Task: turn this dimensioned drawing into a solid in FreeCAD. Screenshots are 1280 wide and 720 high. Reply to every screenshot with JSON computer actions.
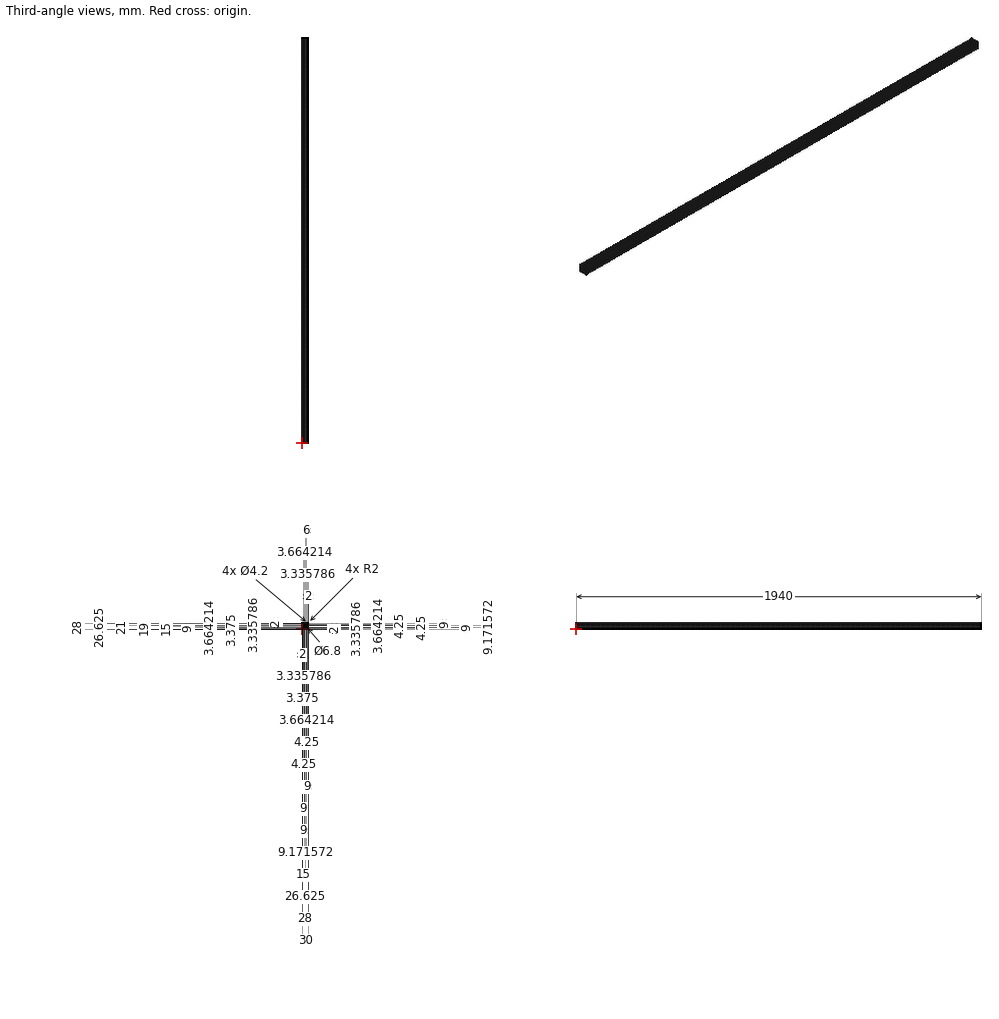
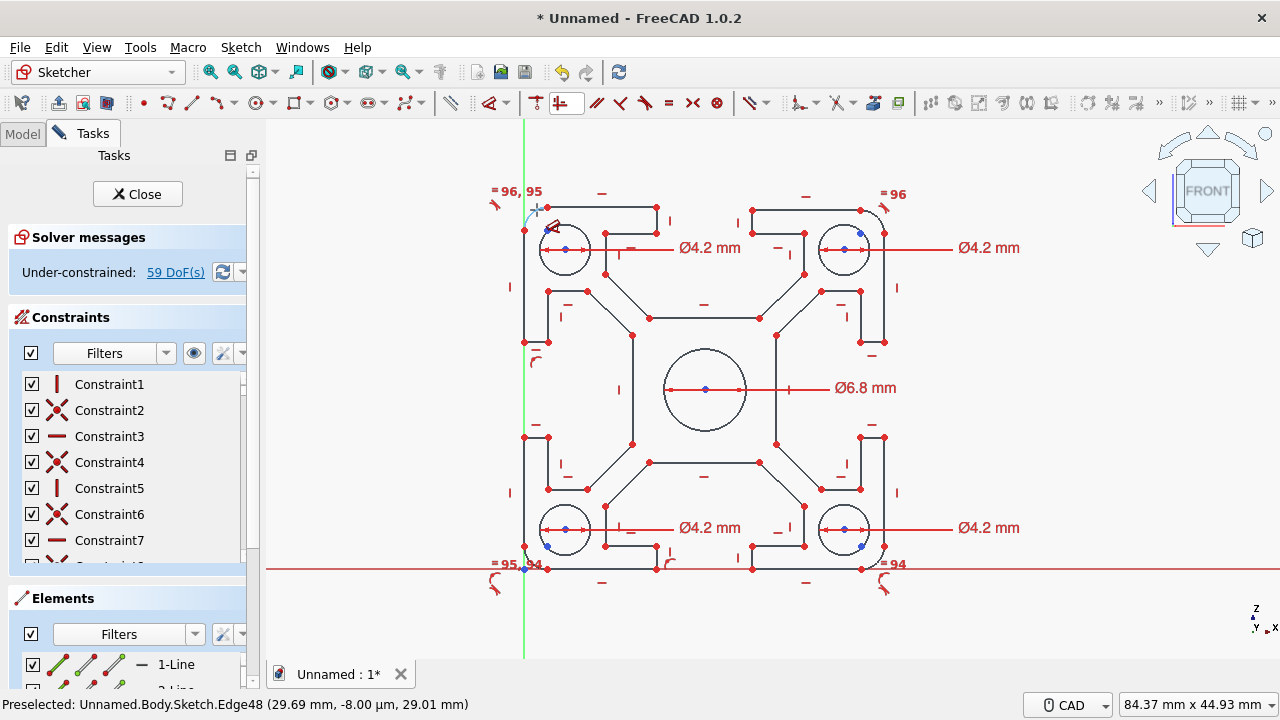
{"action": "scroll", "coordinate": [872, 567], "scroll_direction": "up", "scroll_amount": 3}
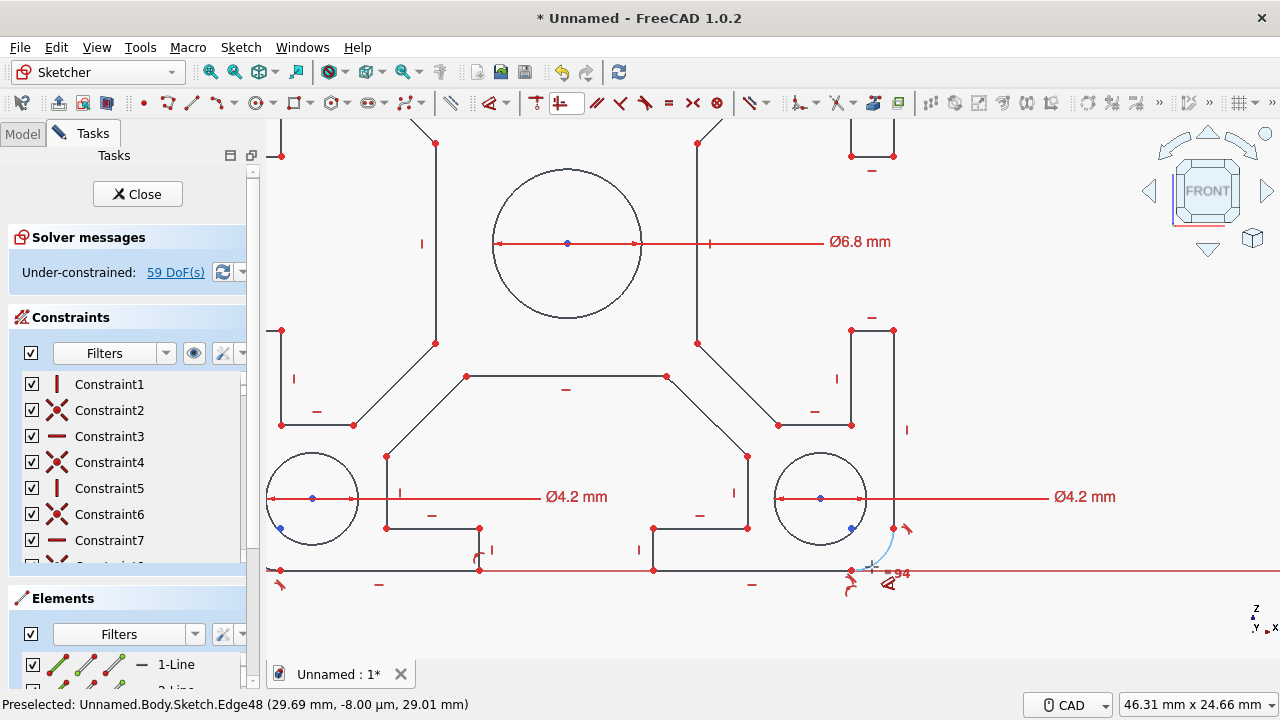
{"action": "left_click", "coordinate": [871, 566]}
{"action": "left_click", "coordinate": [886, 594]}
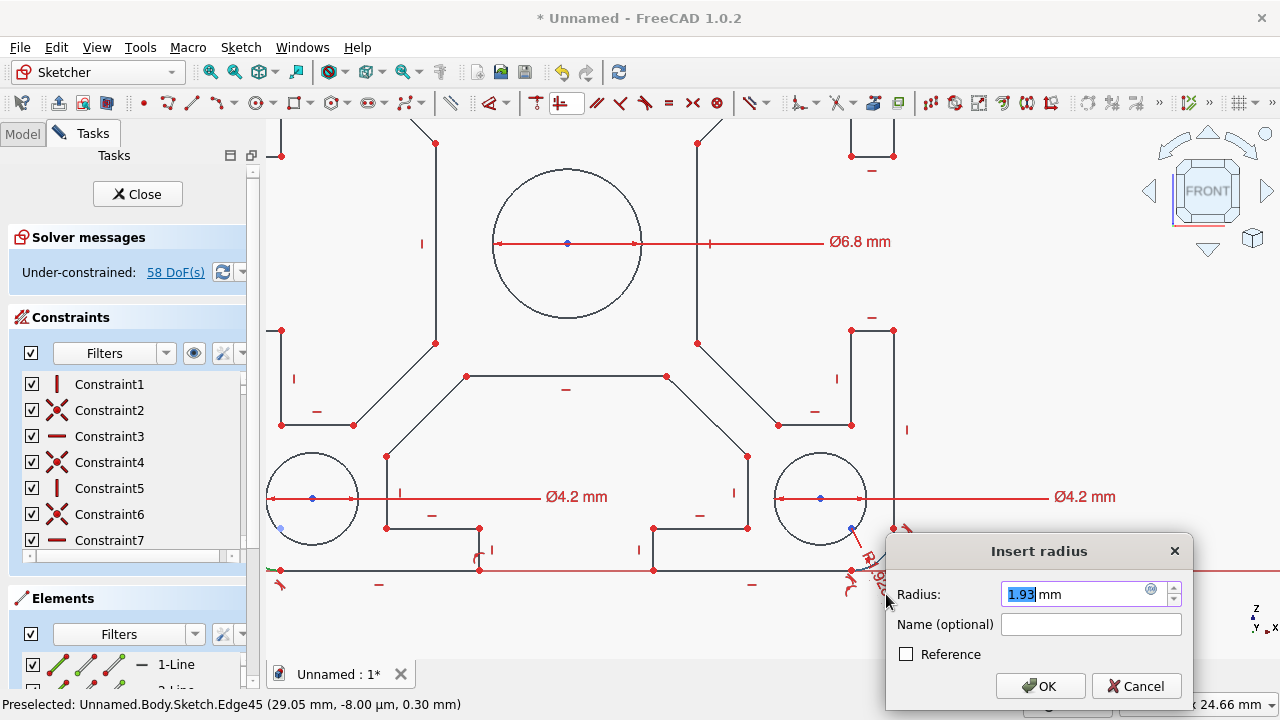
{"action": "type", "text": "2"}
{"action": "key", "text": "Return"}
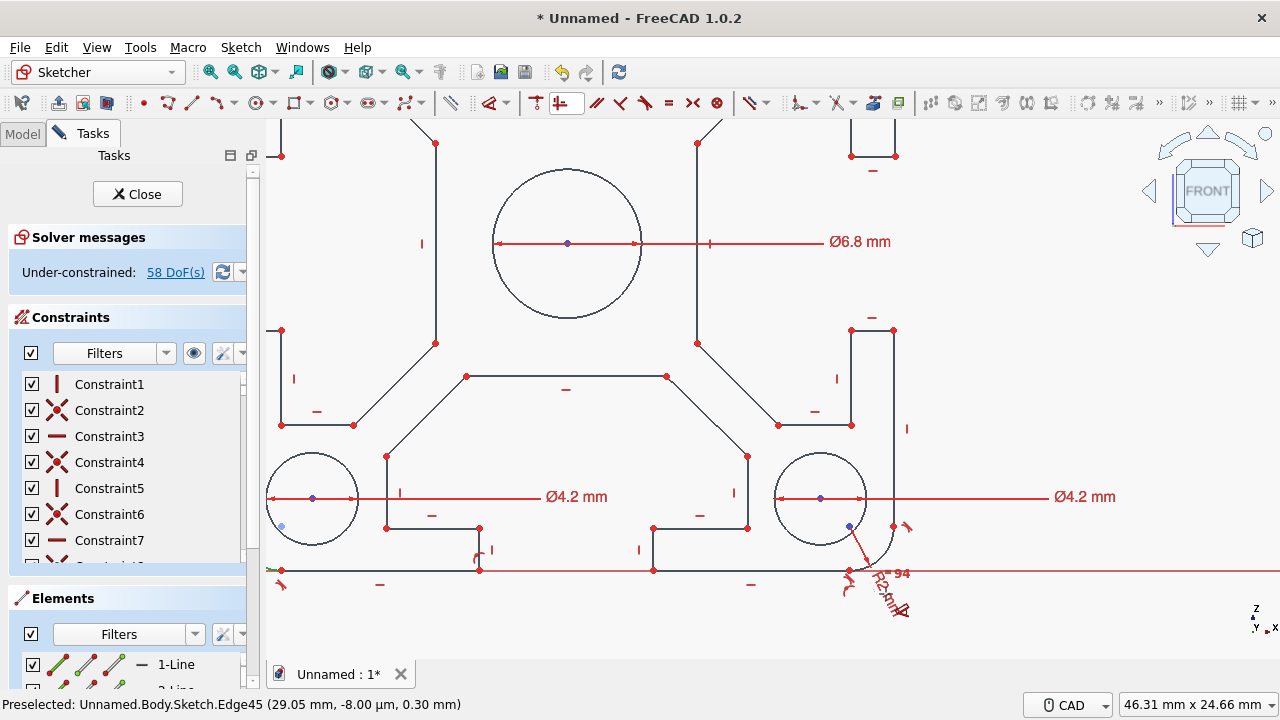
{"action": "scroll", "coordinate": [872, 567], "scroll_direction": "down", "scroll_amount": 3}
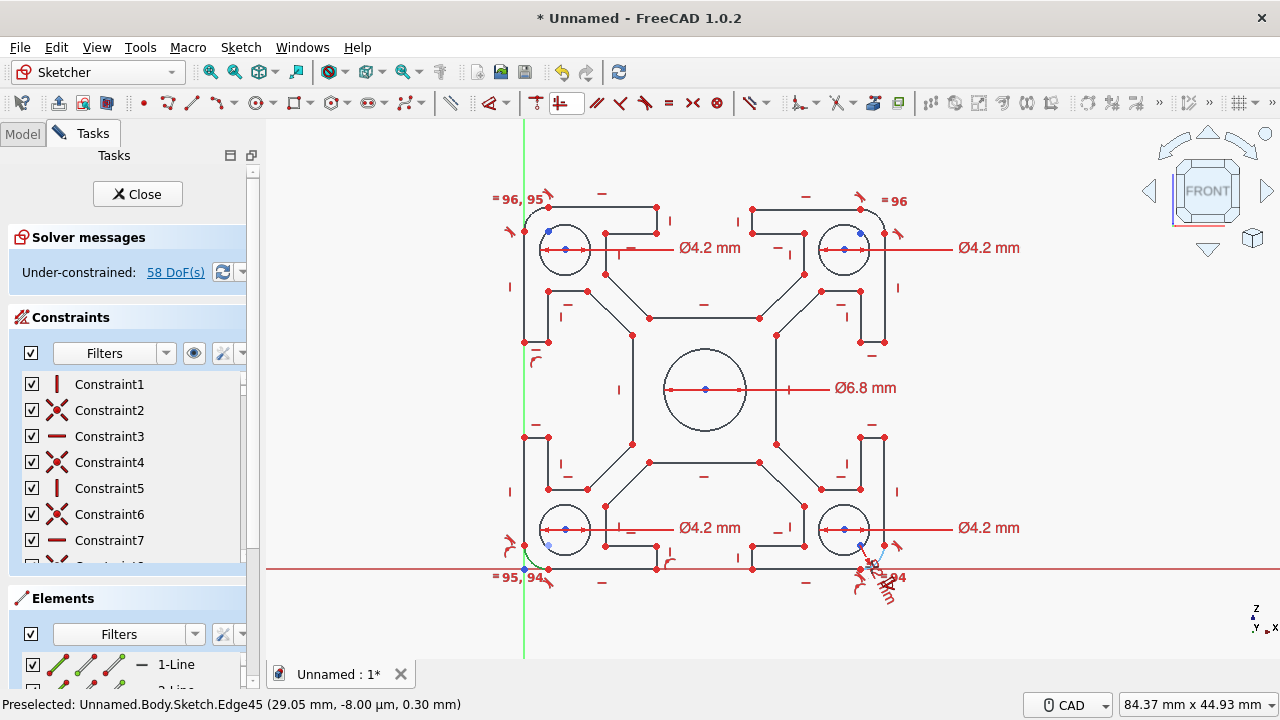
{"action": "left_click", "coordinate": [885, 266]}
{"action": "left_click", "coordinate": [919, 288]}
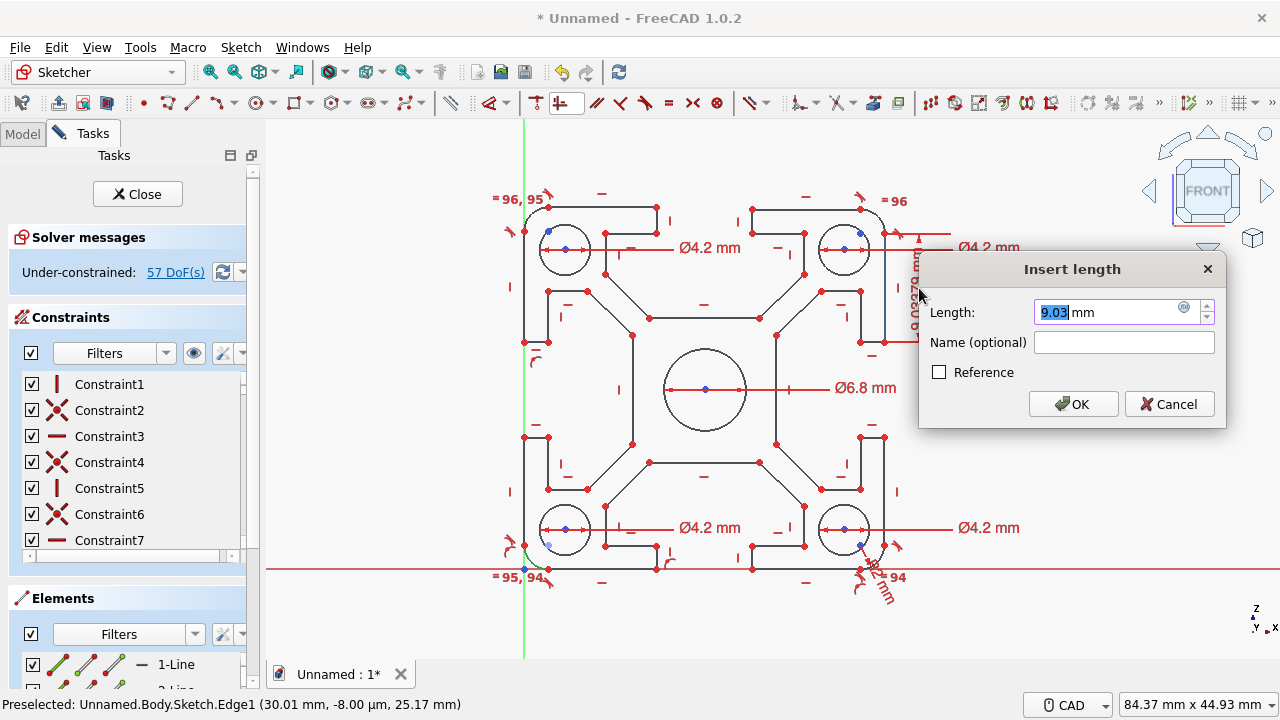
{"action": "type", "text": "9"}
{"action": "key", "text": "Return"}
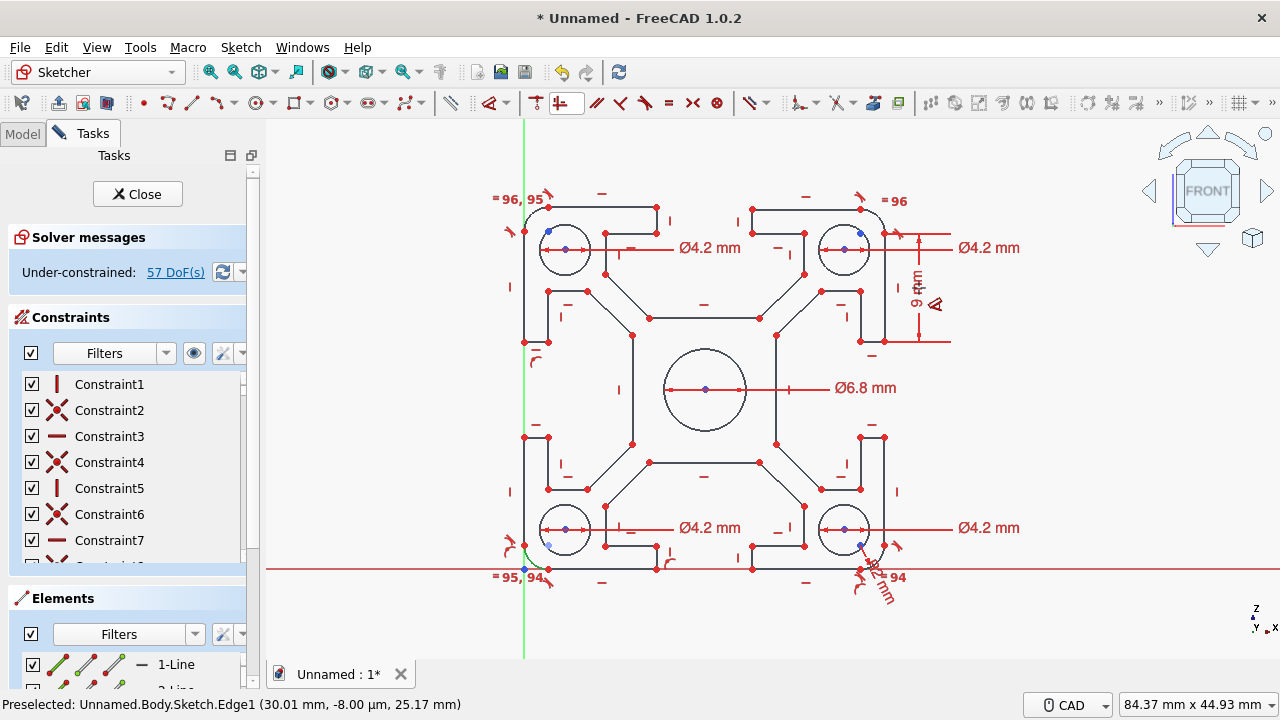
{"action": "scroll", "coordinate": [875, 342], "scroll_direction": "up", "scroll_amount": 3}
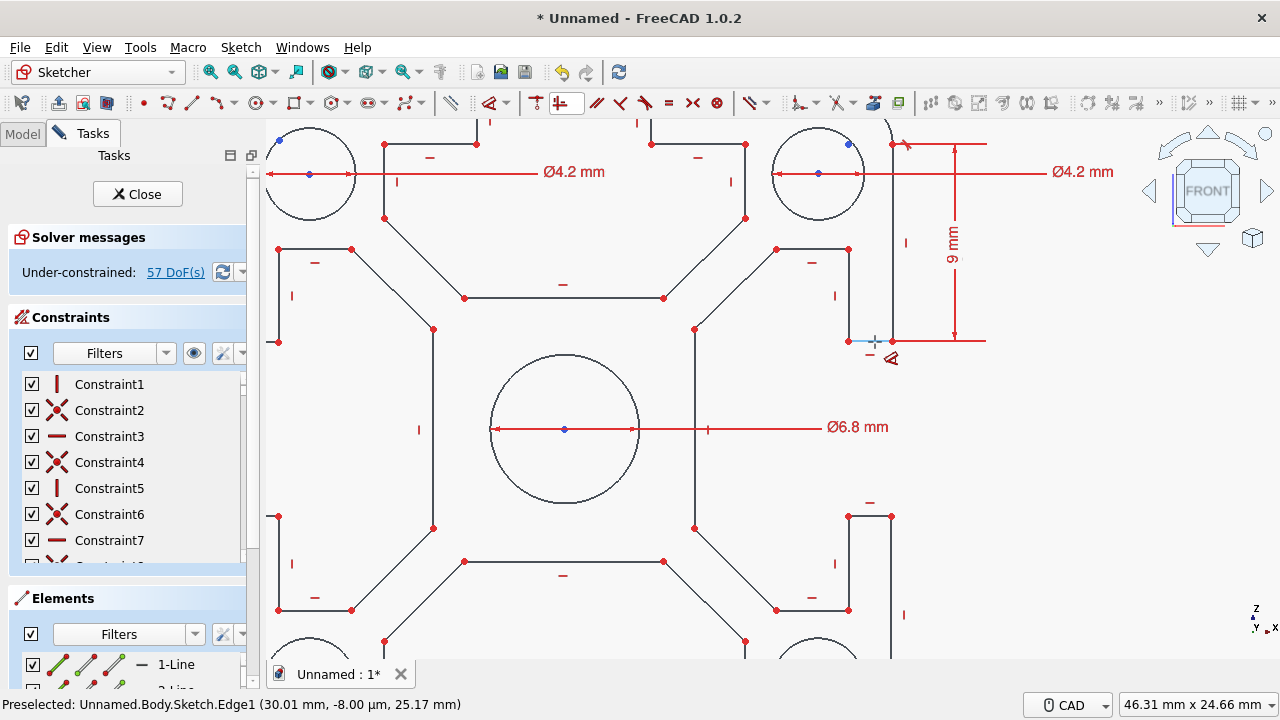
{"action": "left_click", "coordinate": [875, 341]}
{"action": "left_click", "coordinate": [871, 307]}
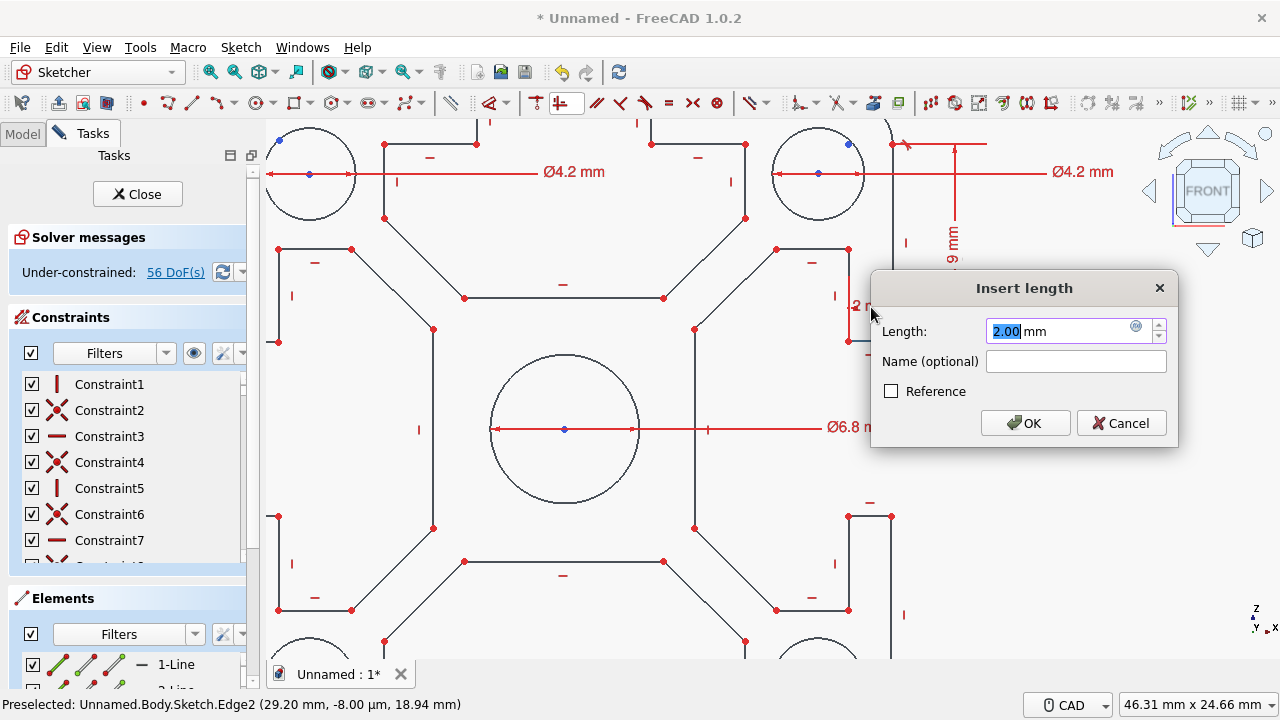
{"action": "type", "text": "2"}
{"action": "key", "text": "Return"}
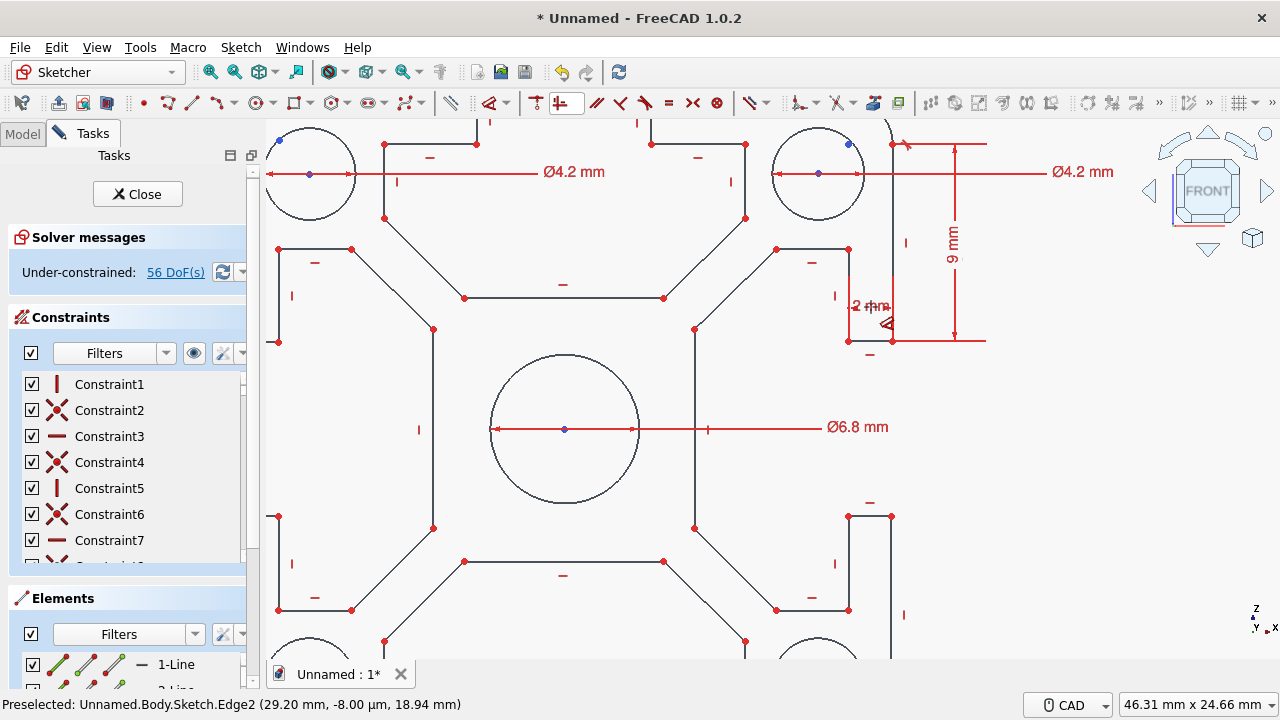
{"action": "left_click", "coordinate": [862, 516]}
{"action": "left_click", "coordinate": [870, 550]}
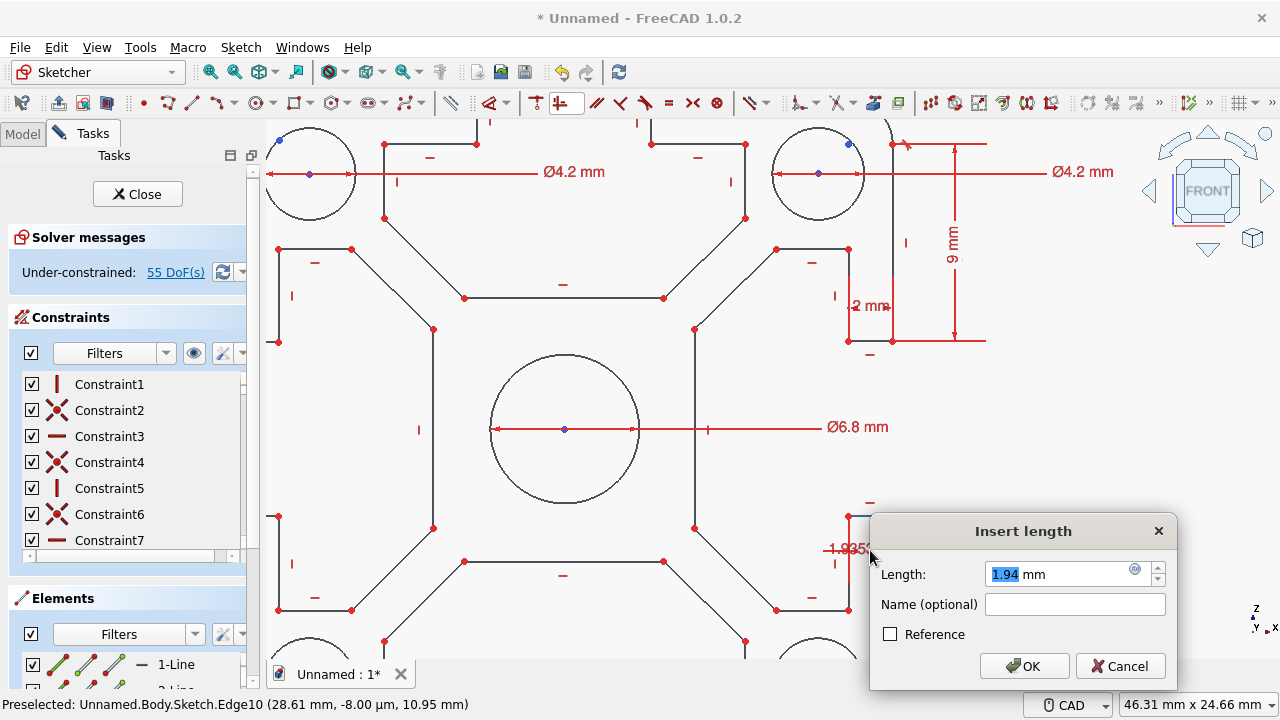
{"action": "type", "text": "2"}
{"action": "key", "text": "Return"}